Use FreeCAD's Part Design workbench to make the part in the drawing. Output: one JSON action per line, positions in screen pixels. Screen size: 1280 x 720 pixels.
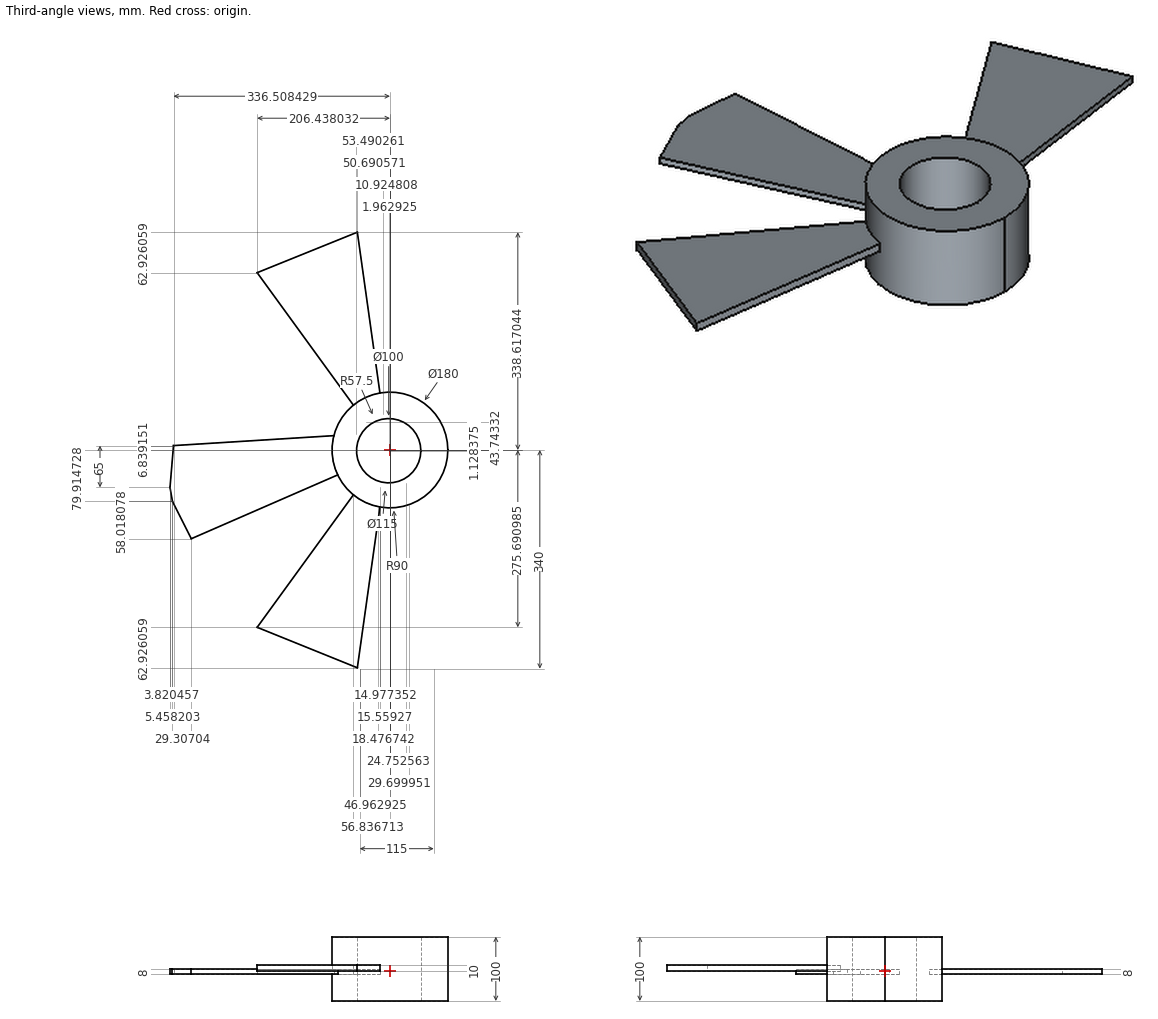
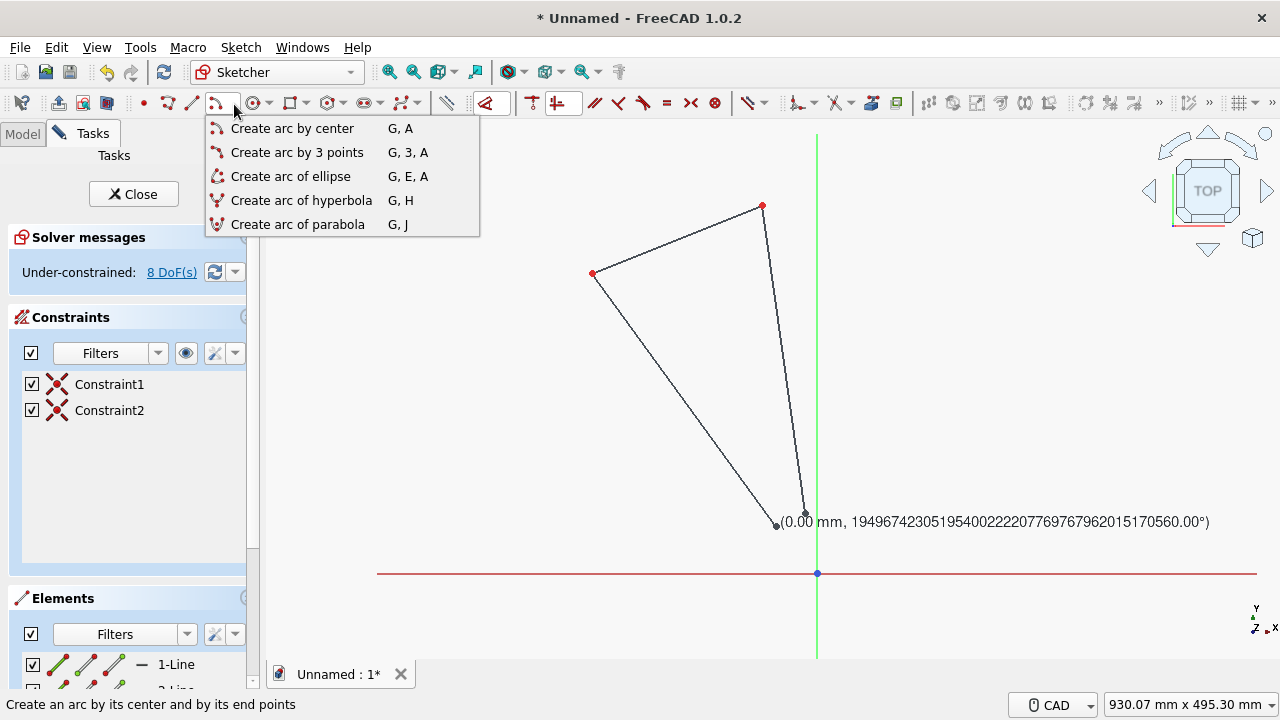
{"action": "left_click", "coordinate": [342, 152]}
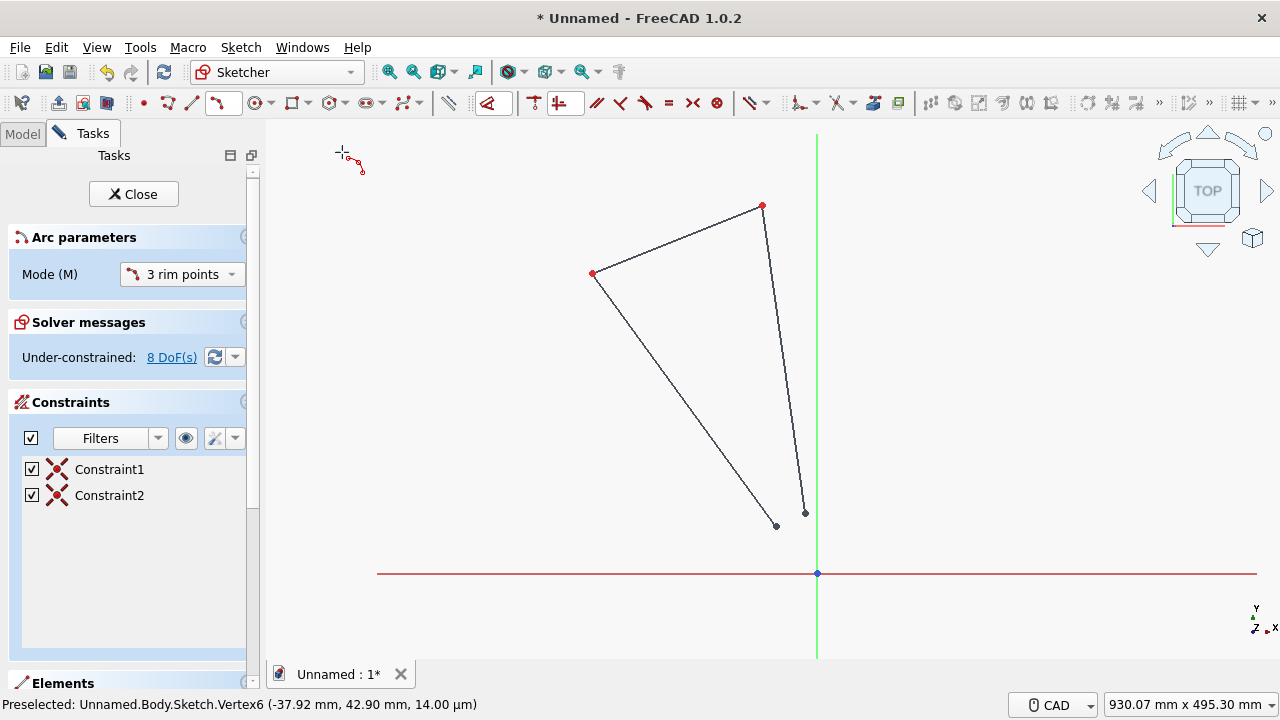
{"action": "left_click", "coordinate": [776, 527]}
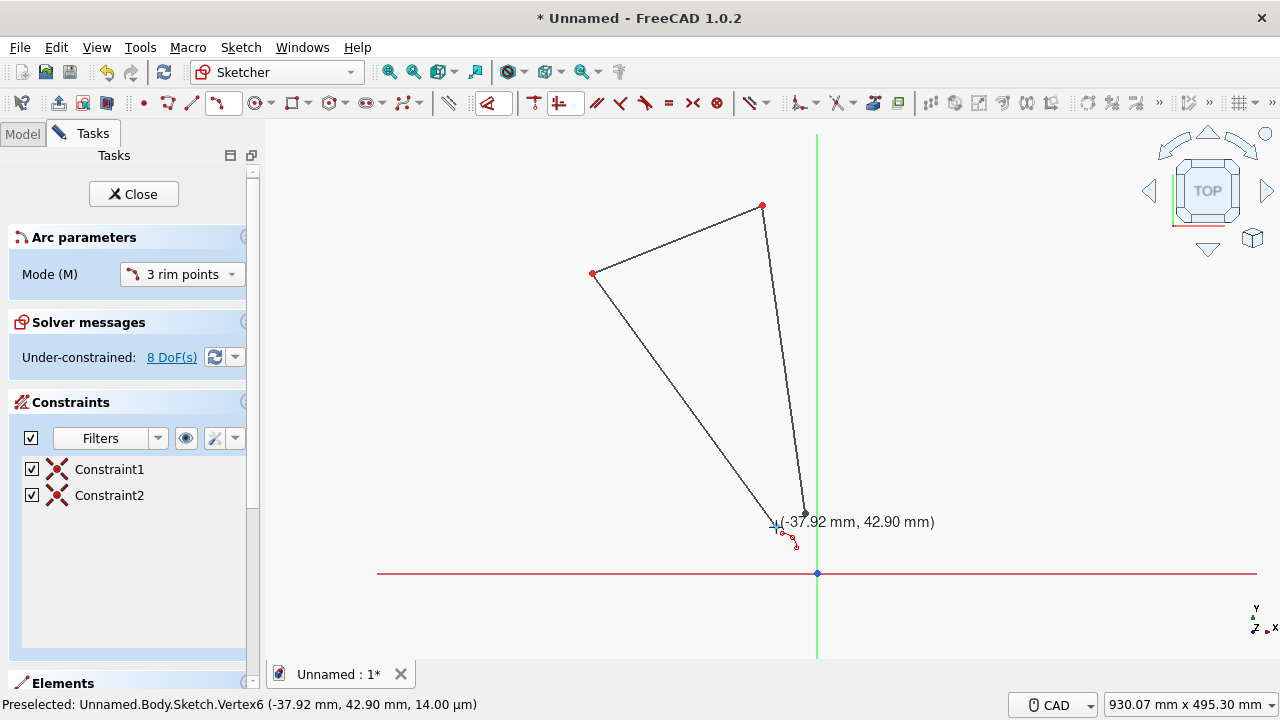
{"action": "scroll", "coordinate": [805, 513], "scroll_direction": "up", "scroll_amount": 2}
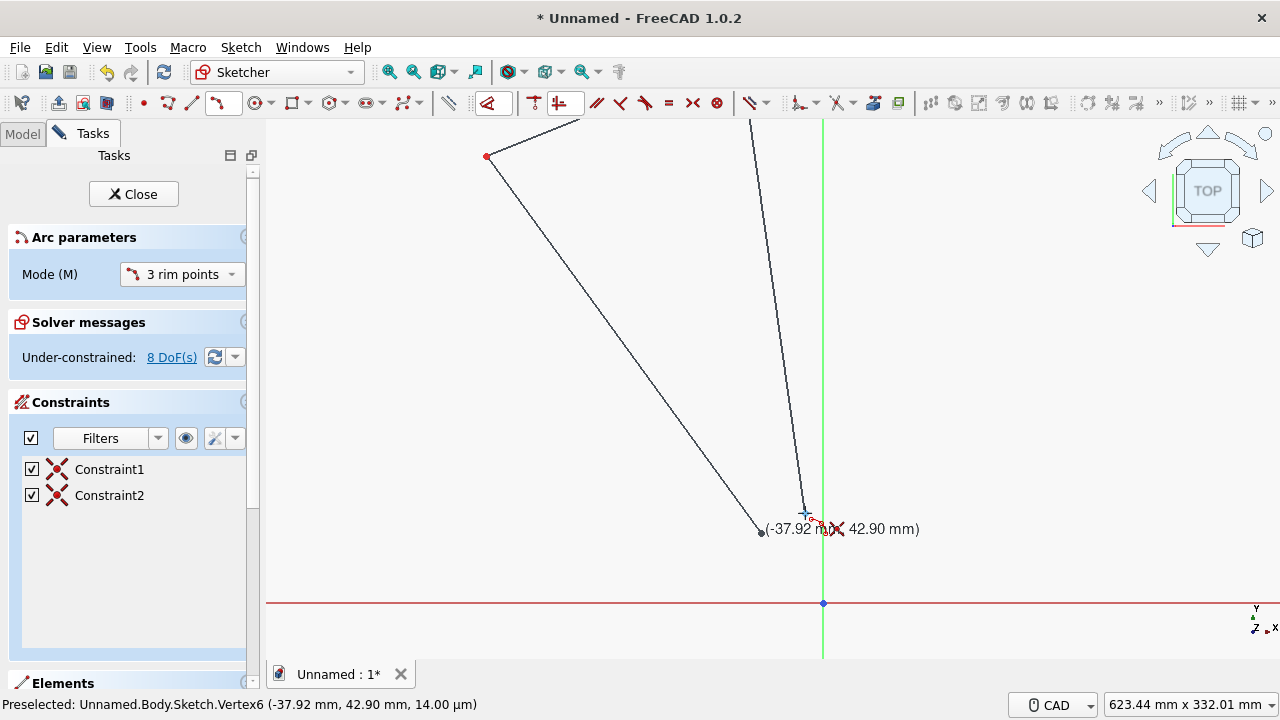
{"action": "left_click", "coordinate": [805, 514]}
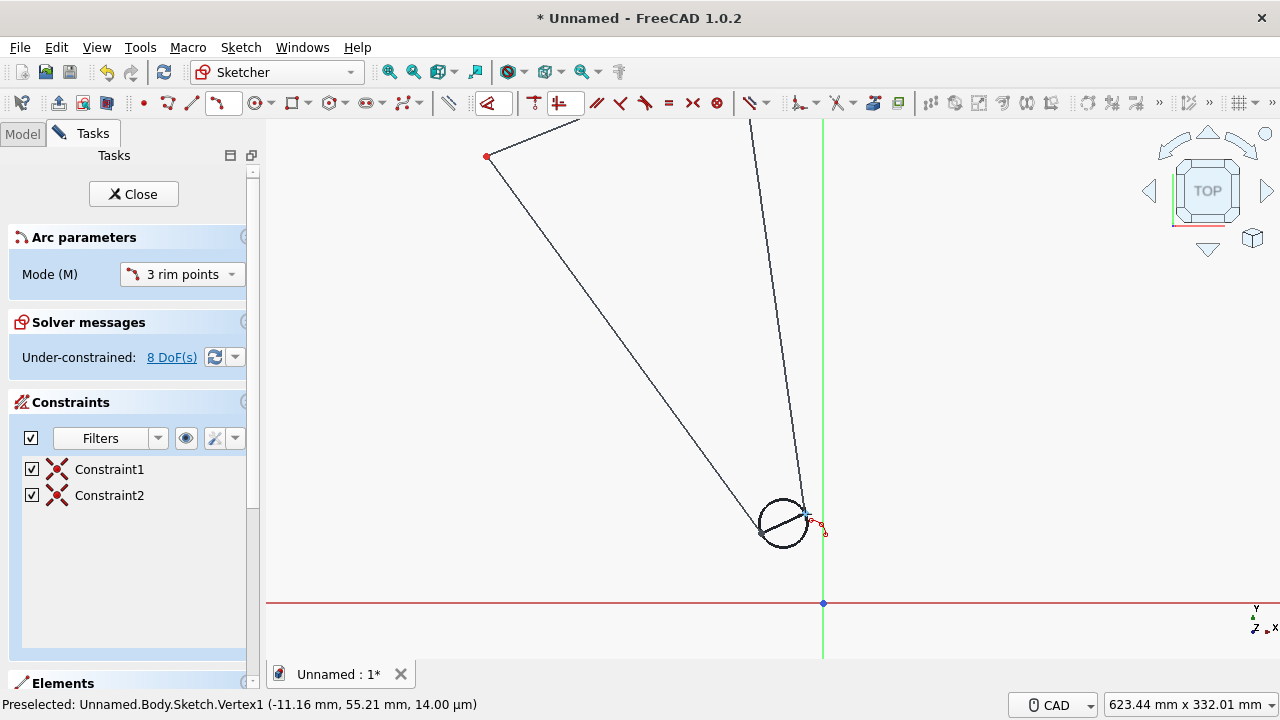
{"action": "scroll", "coordinate": [782, 520], "scroll_direction": "up", "scroll_amount": 9}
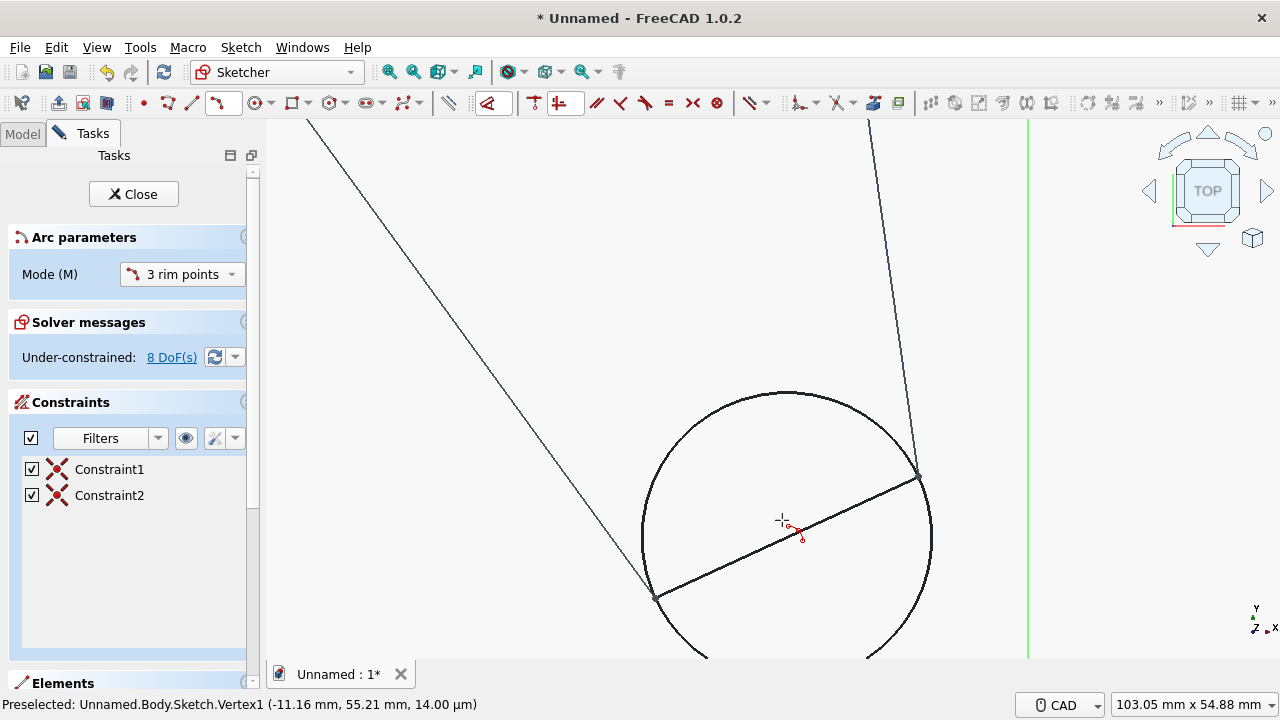
{"action": "left_click", "coordinate": [780, 514]}
{"action": "key", "text": "Escape"}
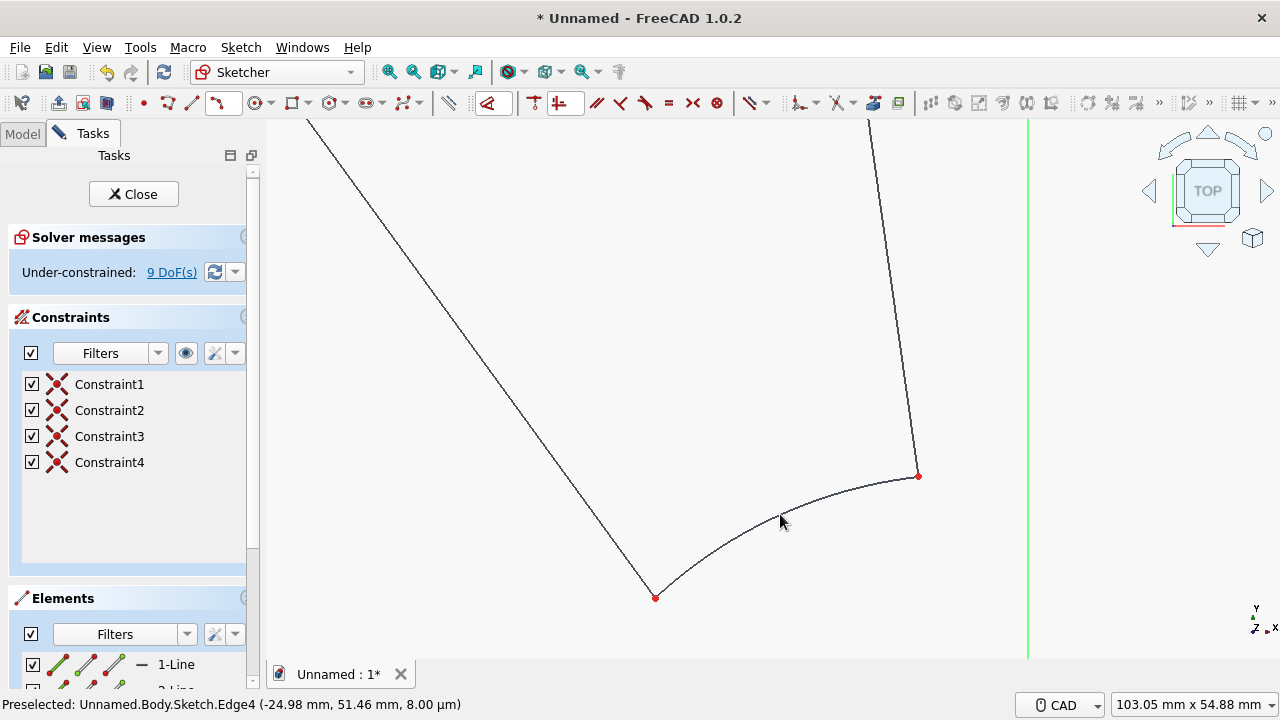
{"action": "left_click", "coordinate": [488, 104]}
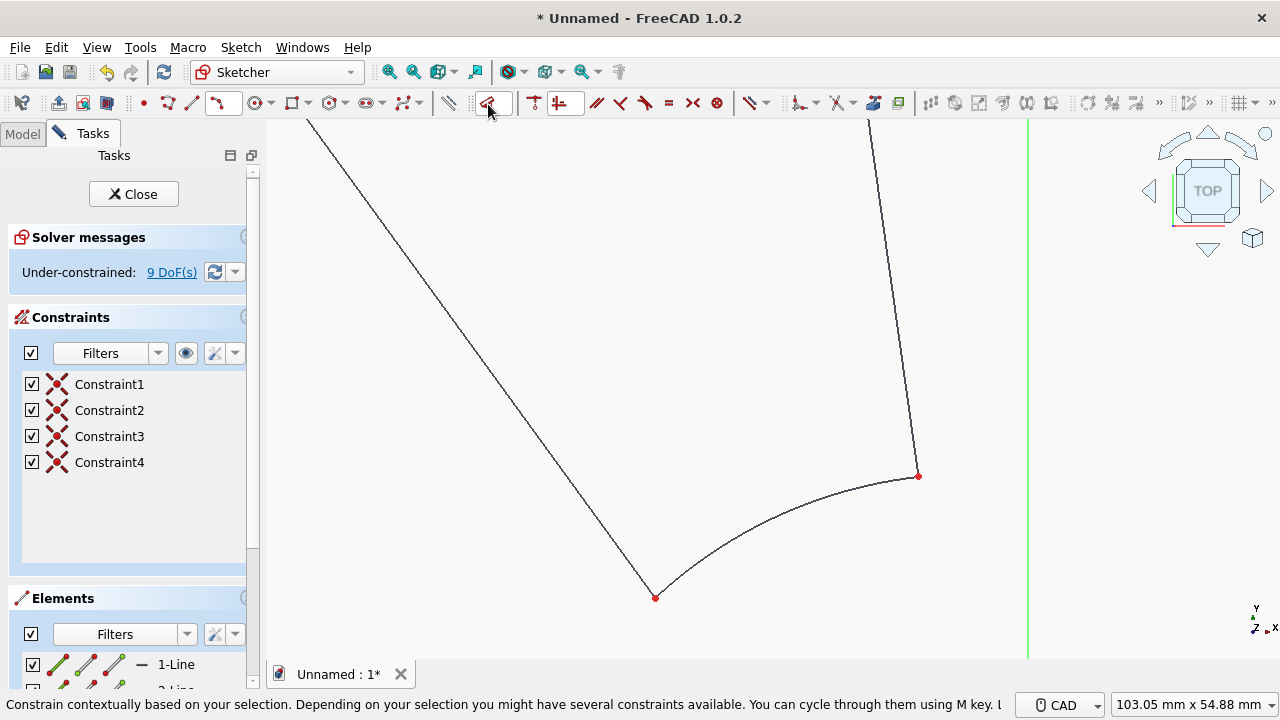
{"action": "scroll", "coordinate": [791, 518], "scroll_direction": "down", "scroll_amount": 11}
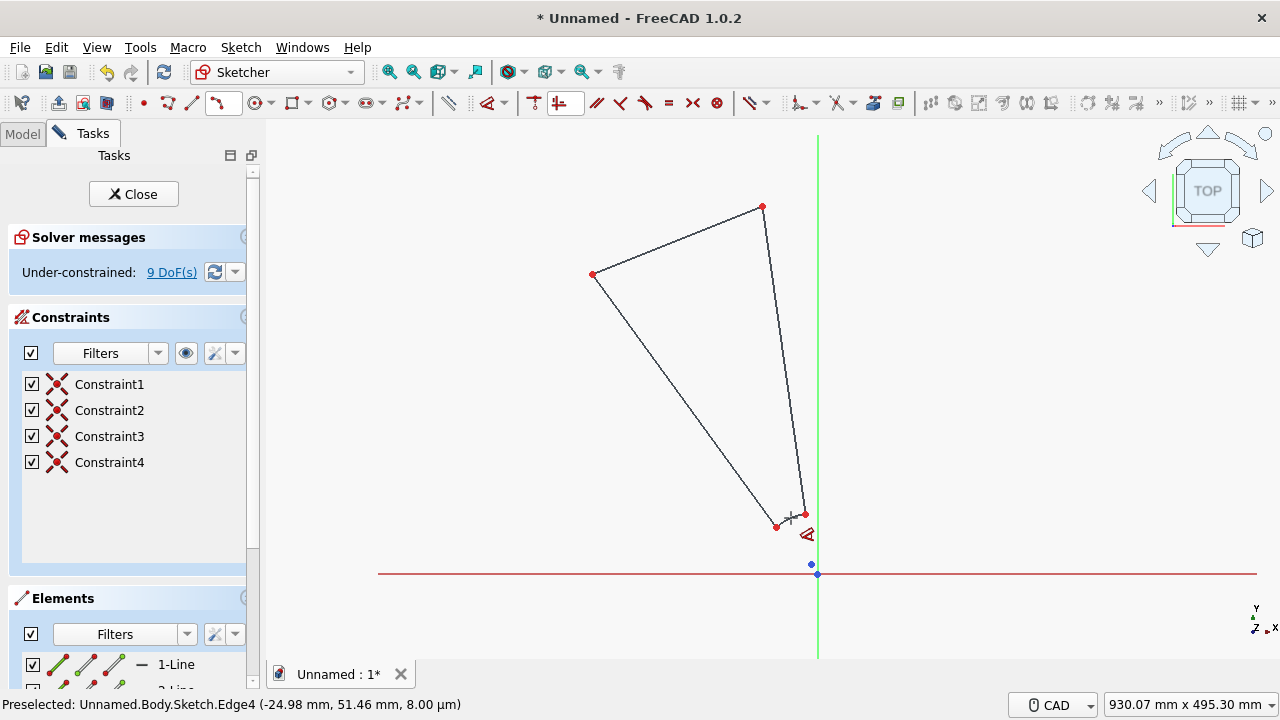
{"action": "scroll", "coordinate": [796, 516], "scroll_direction": "up", "scroll_amount": 2}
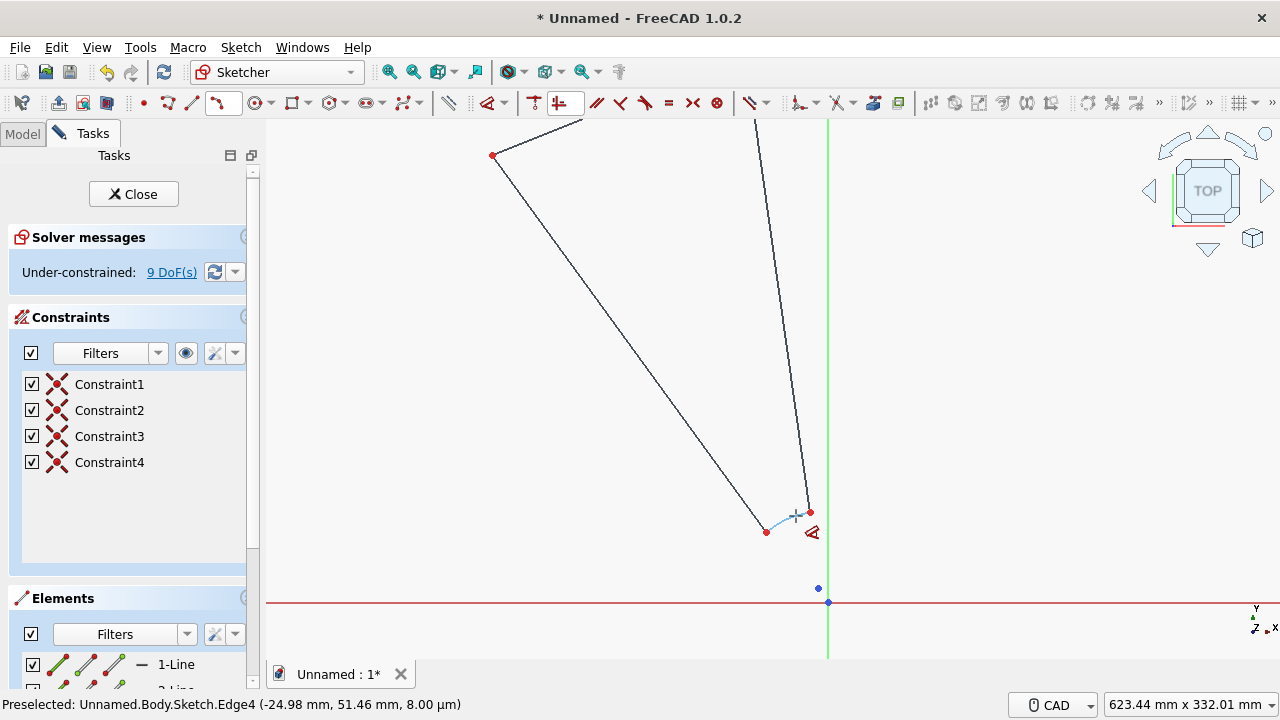
{"action": "left_click", "coordinate": [796, 516]}
{"action": "left_click", "coordinate": [787, 485]}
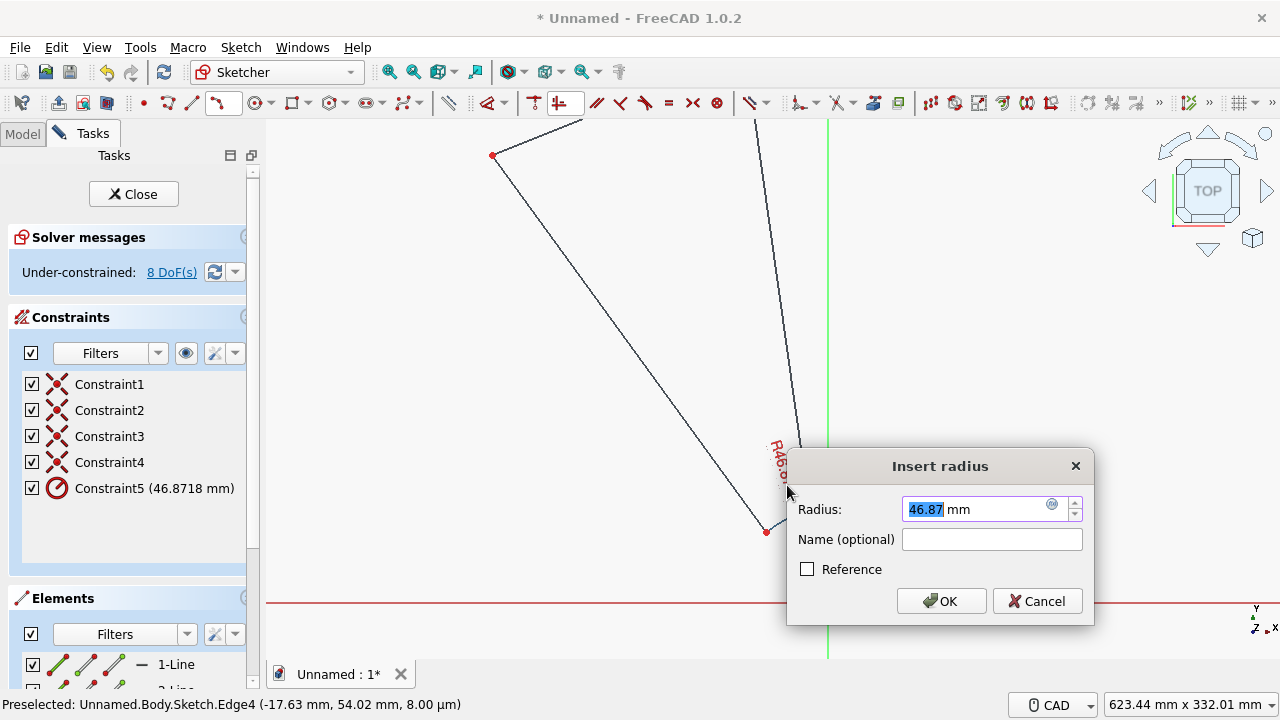
{"action": "type", "text": "57.5"}
{"action": "key", "text": "Return"}